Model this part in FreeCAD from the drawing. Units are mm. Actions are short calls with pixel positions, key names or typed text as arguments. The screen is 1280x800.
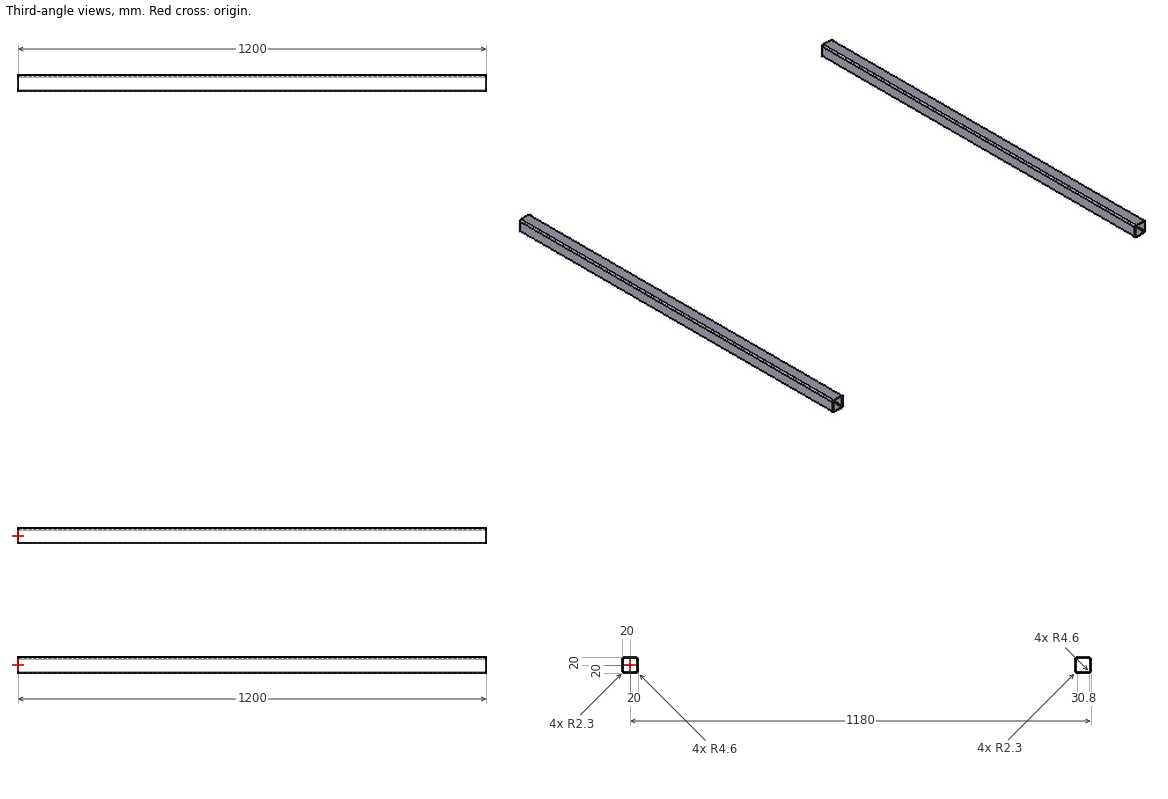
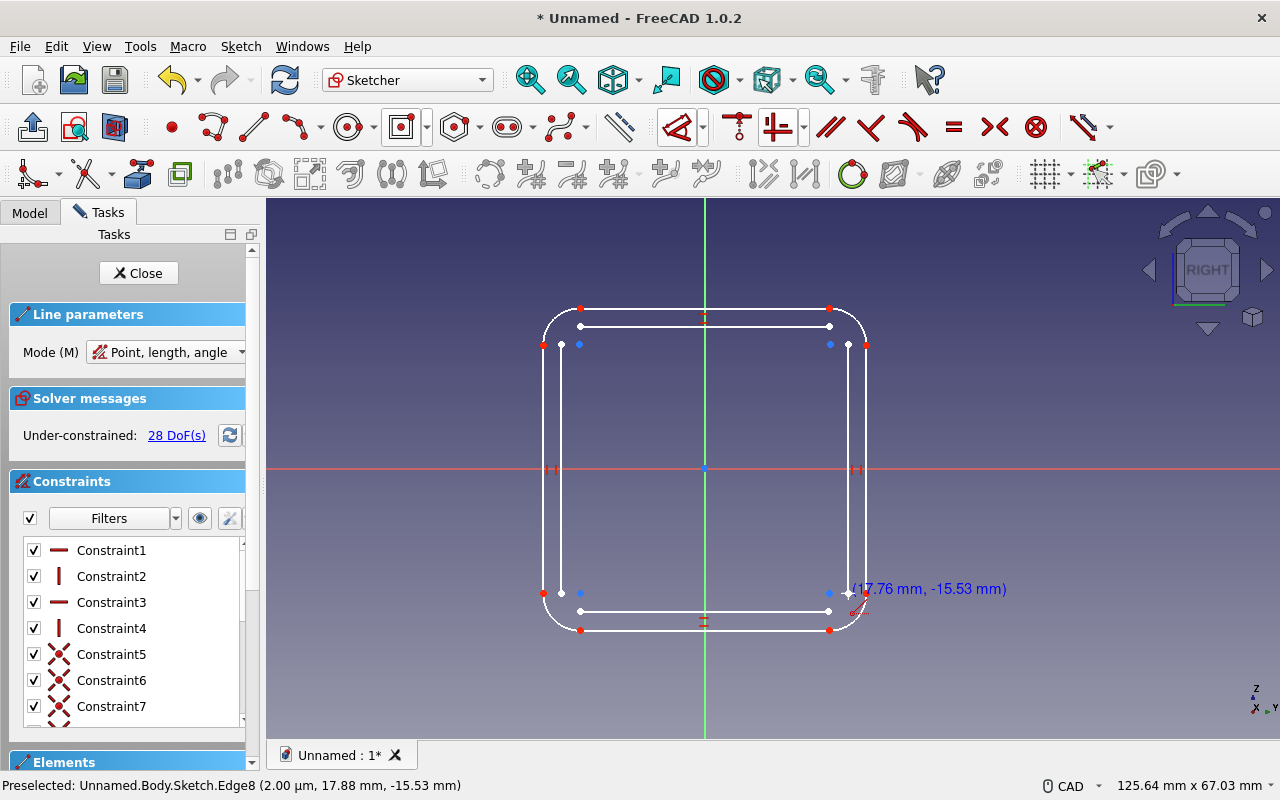
key(g)
key(3)
key(a)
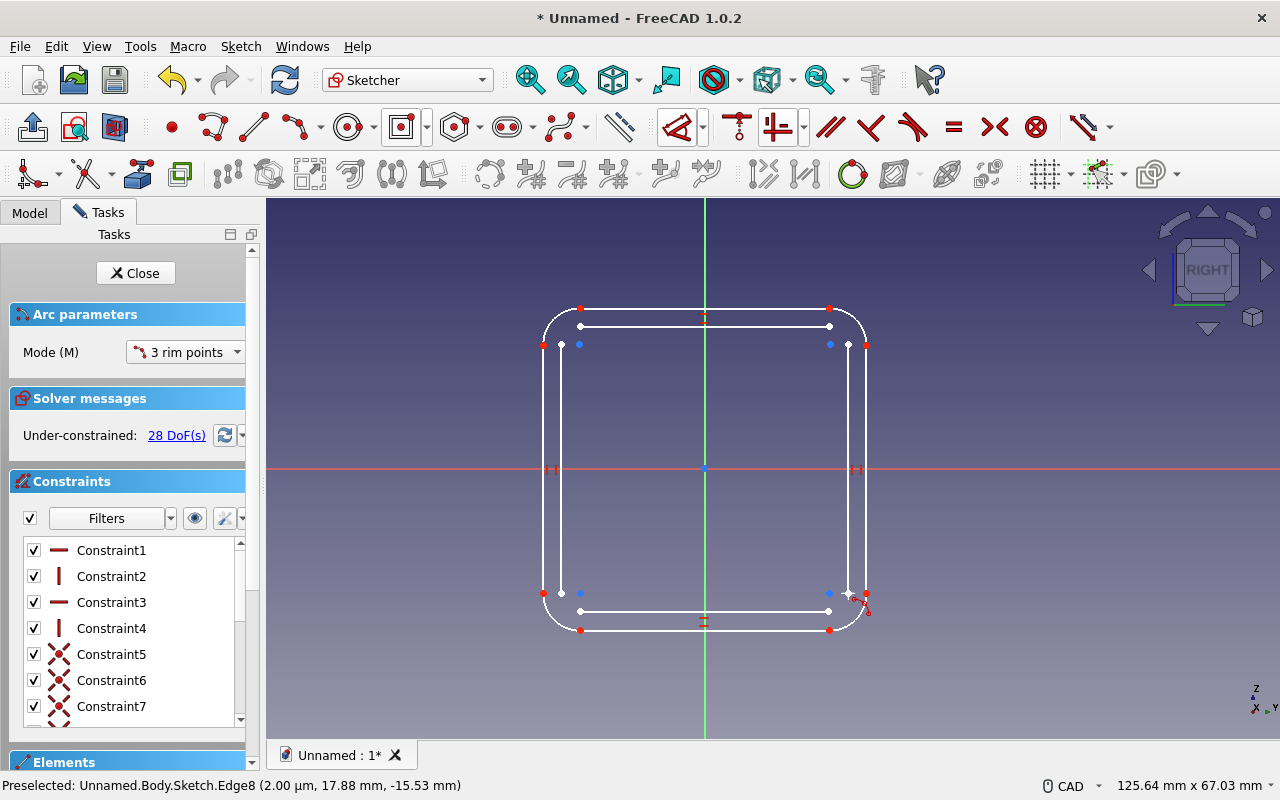
click(580, 612)
click(561, 594)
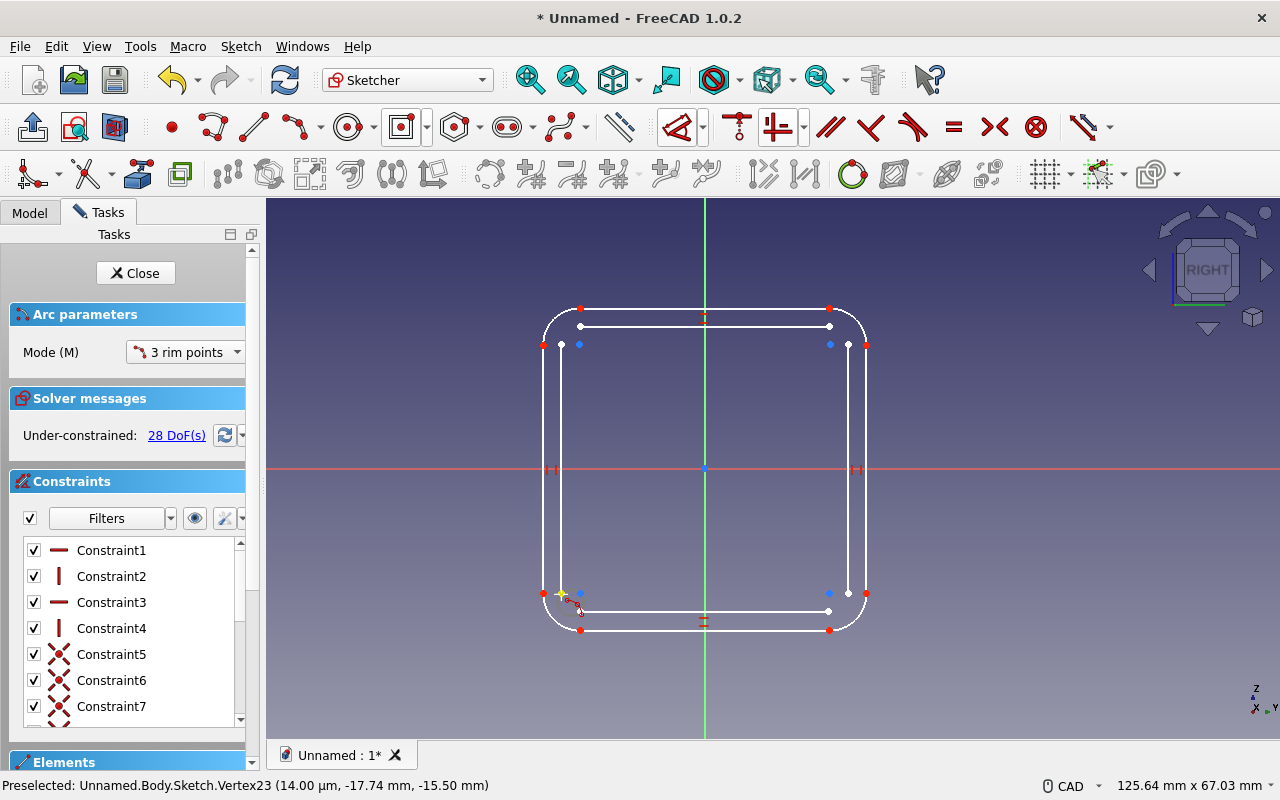
scroll(567, 606, up, 6)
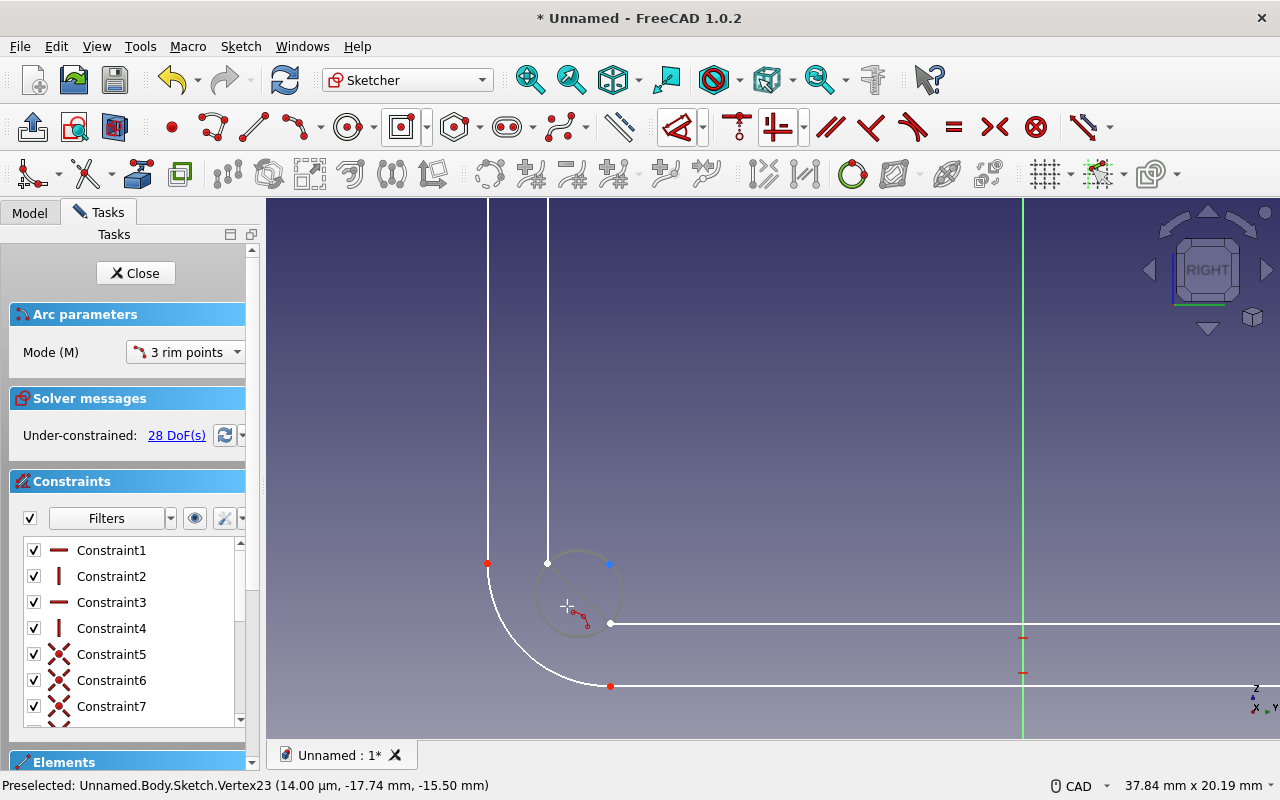
click(567, 605)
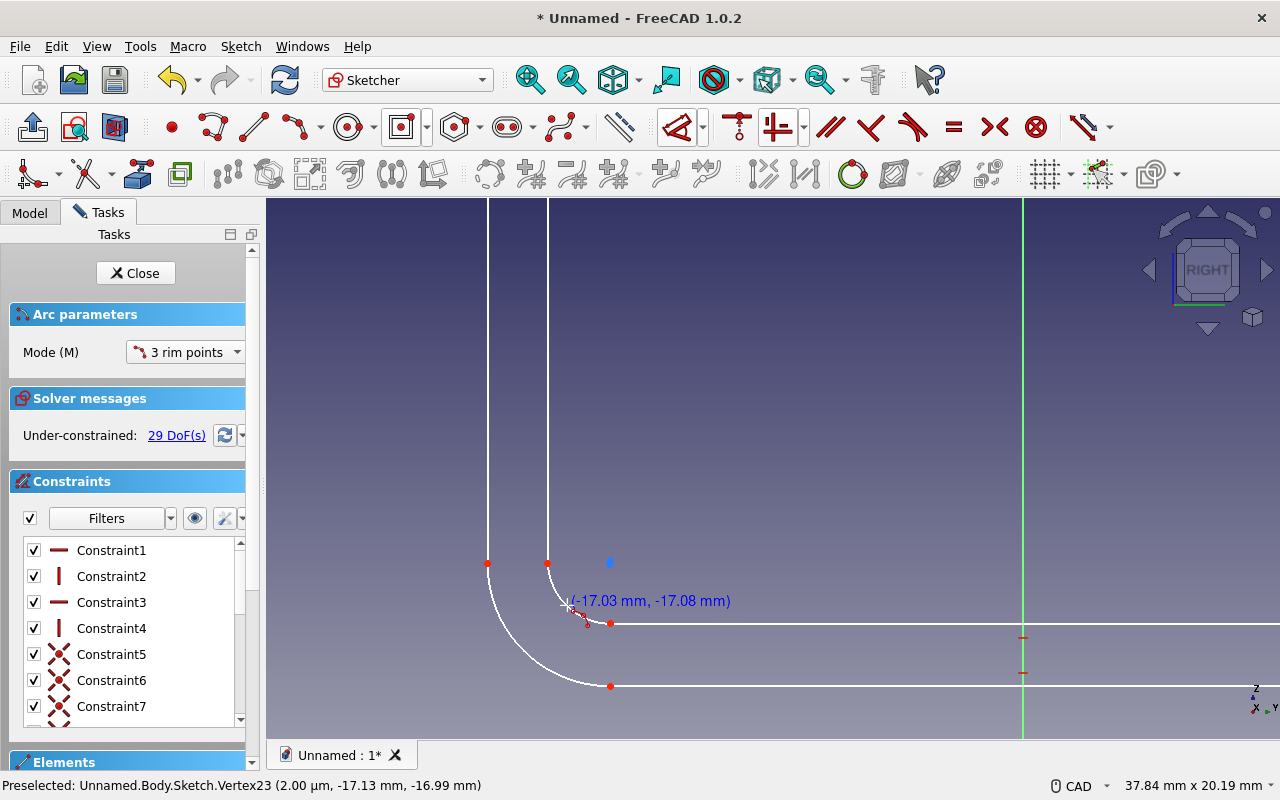
scroll(567, 607, down, 6)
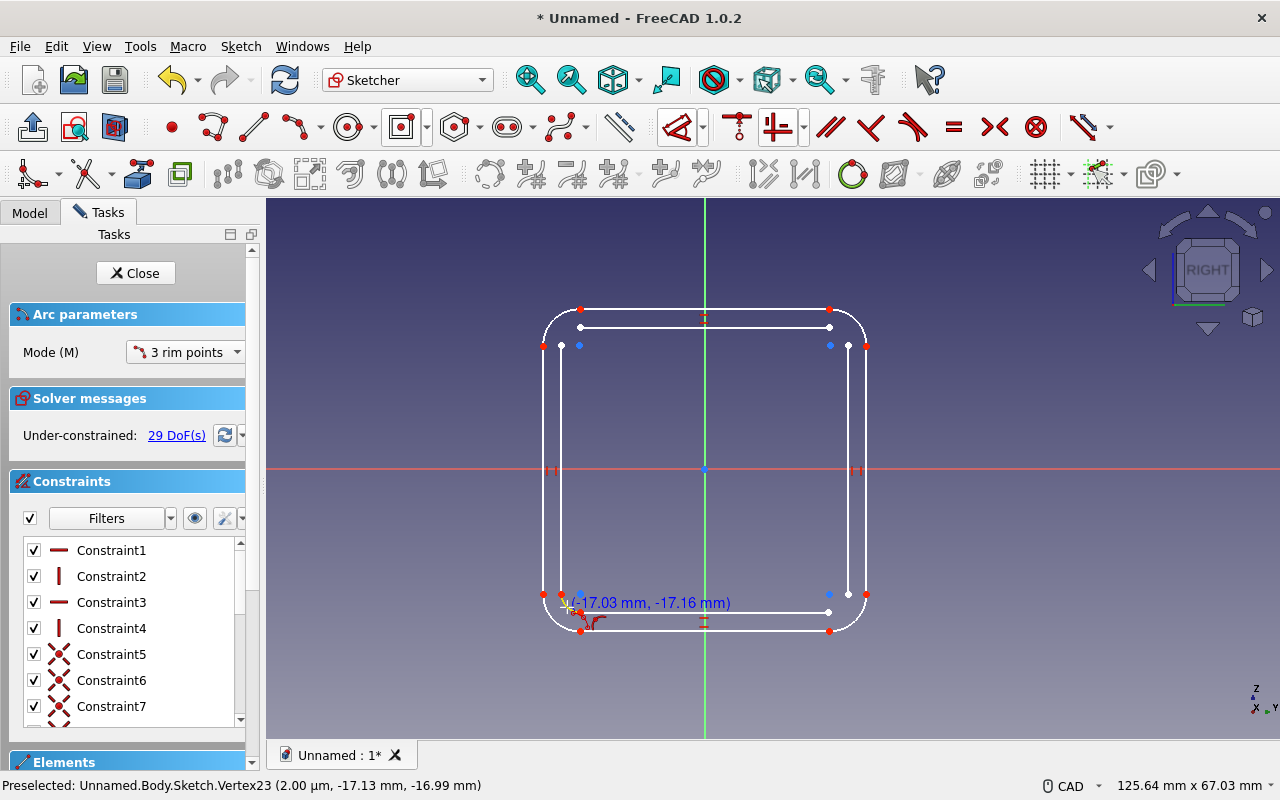
click(561, 346)
click(580, 328)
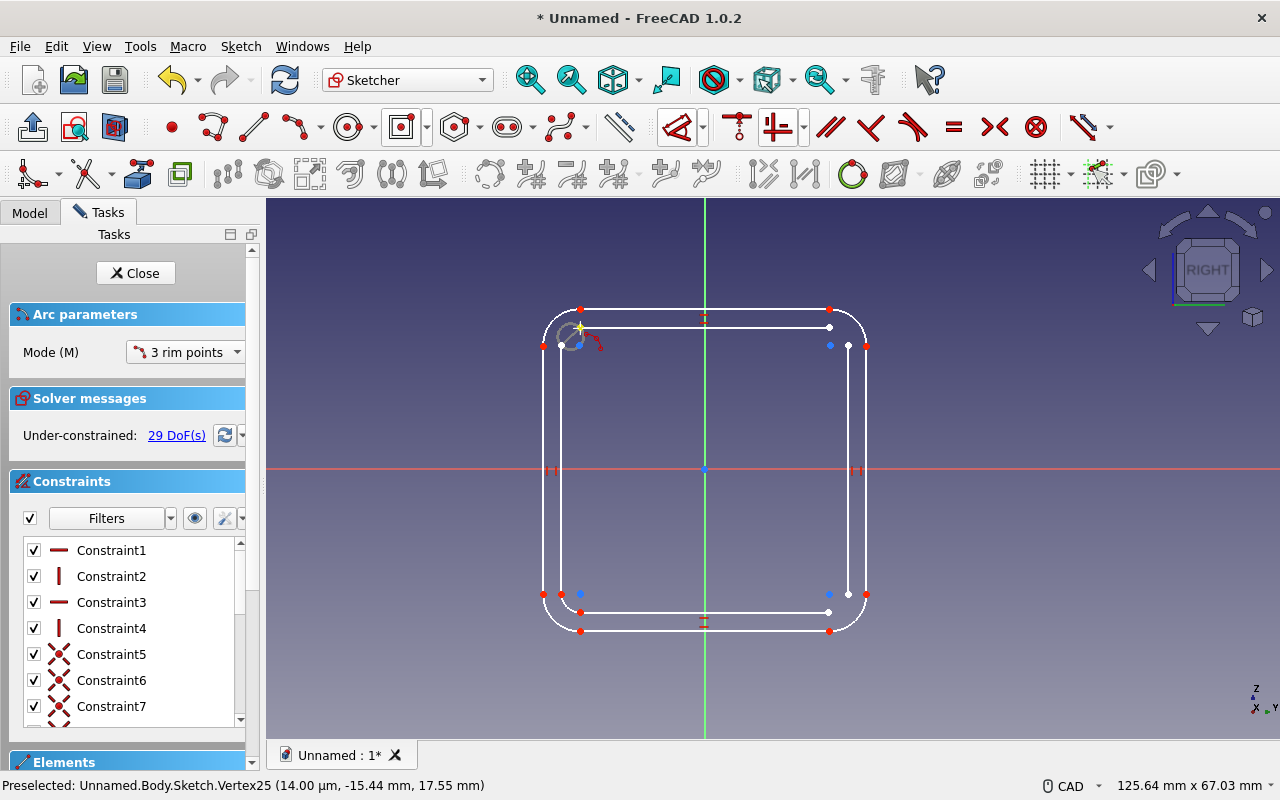
scroll(567, 332, up, 6)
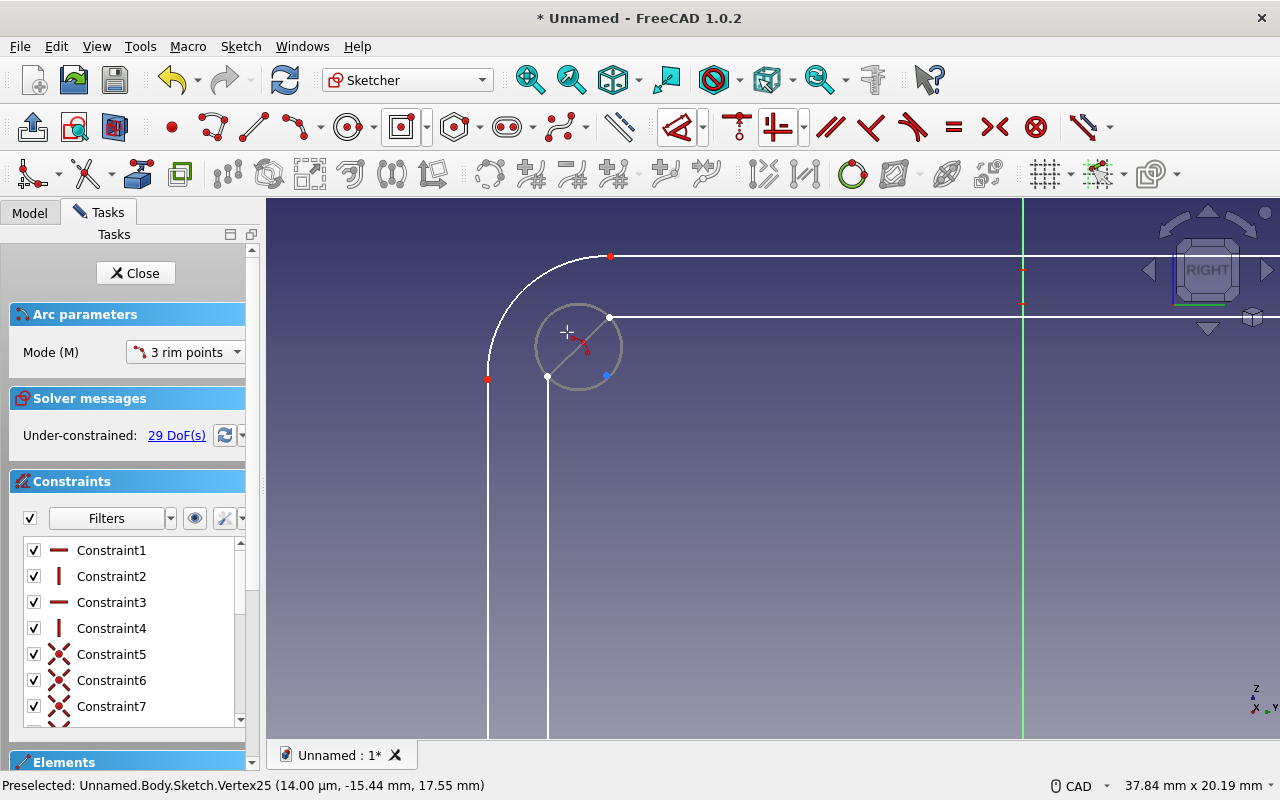
click(567, 331)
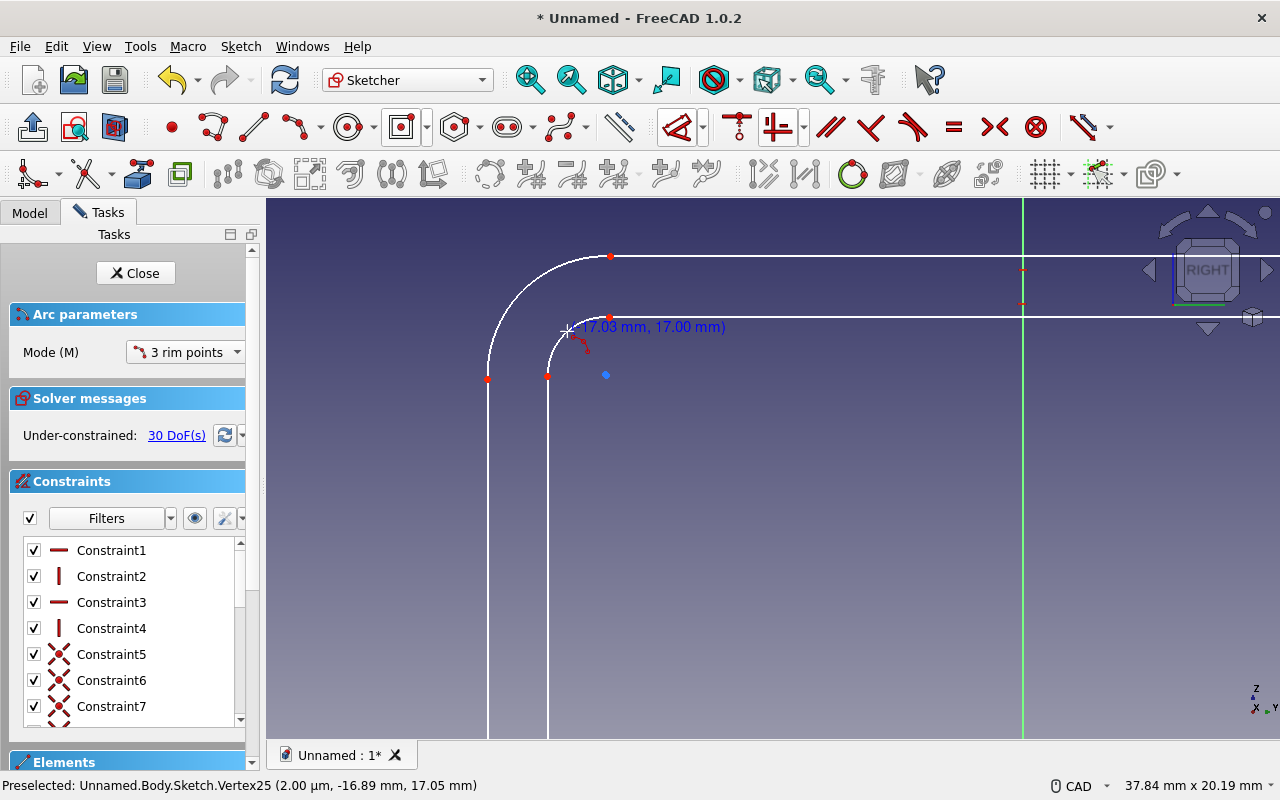
scroll(567, 331, down, 6)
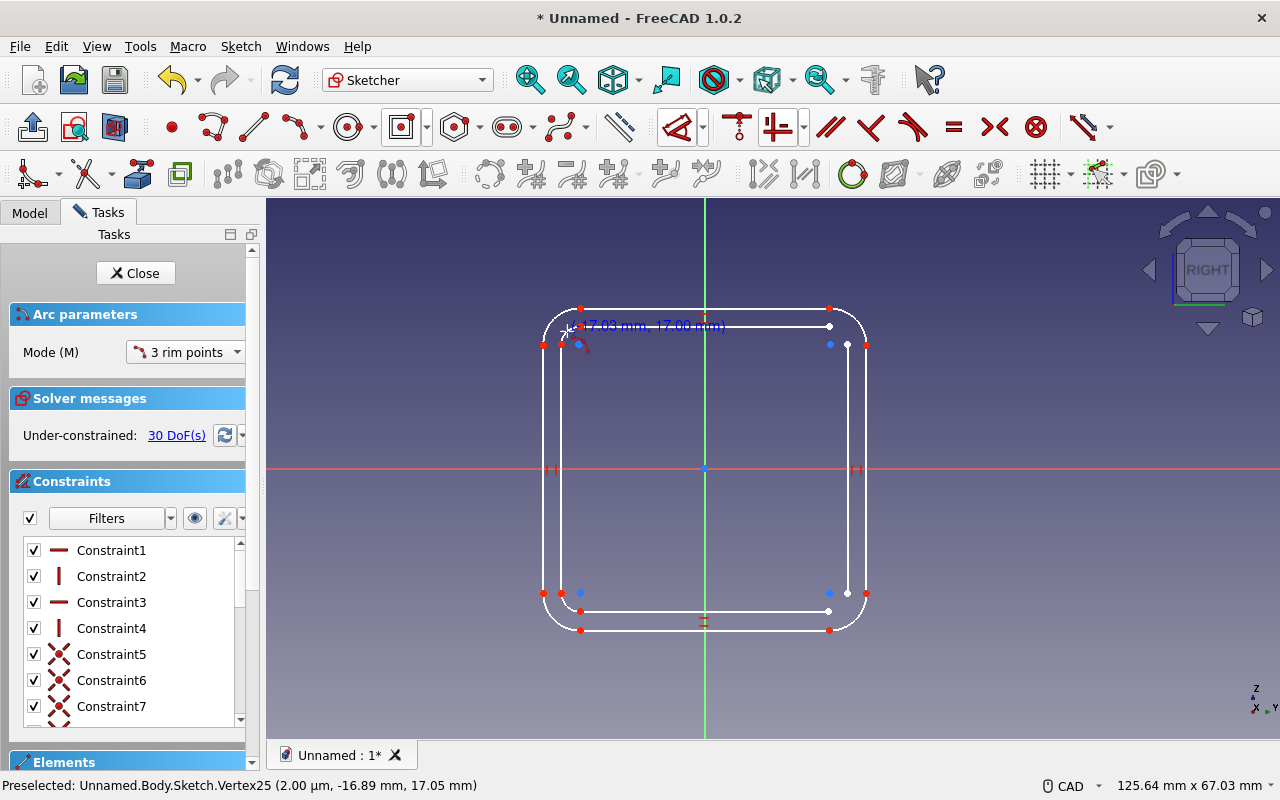
click(829, 327)
click(848, 345)